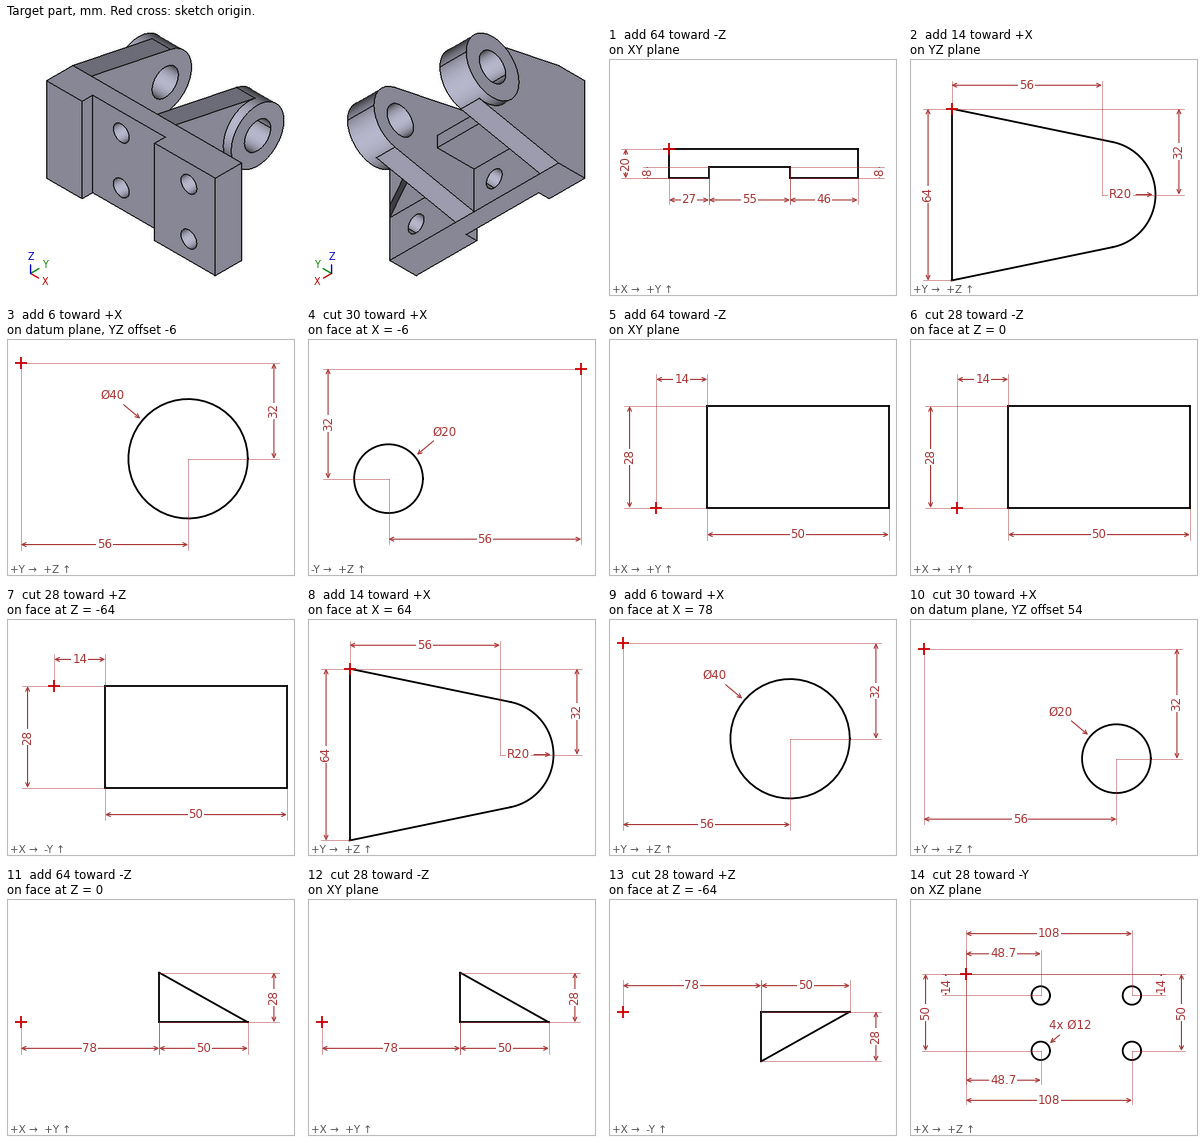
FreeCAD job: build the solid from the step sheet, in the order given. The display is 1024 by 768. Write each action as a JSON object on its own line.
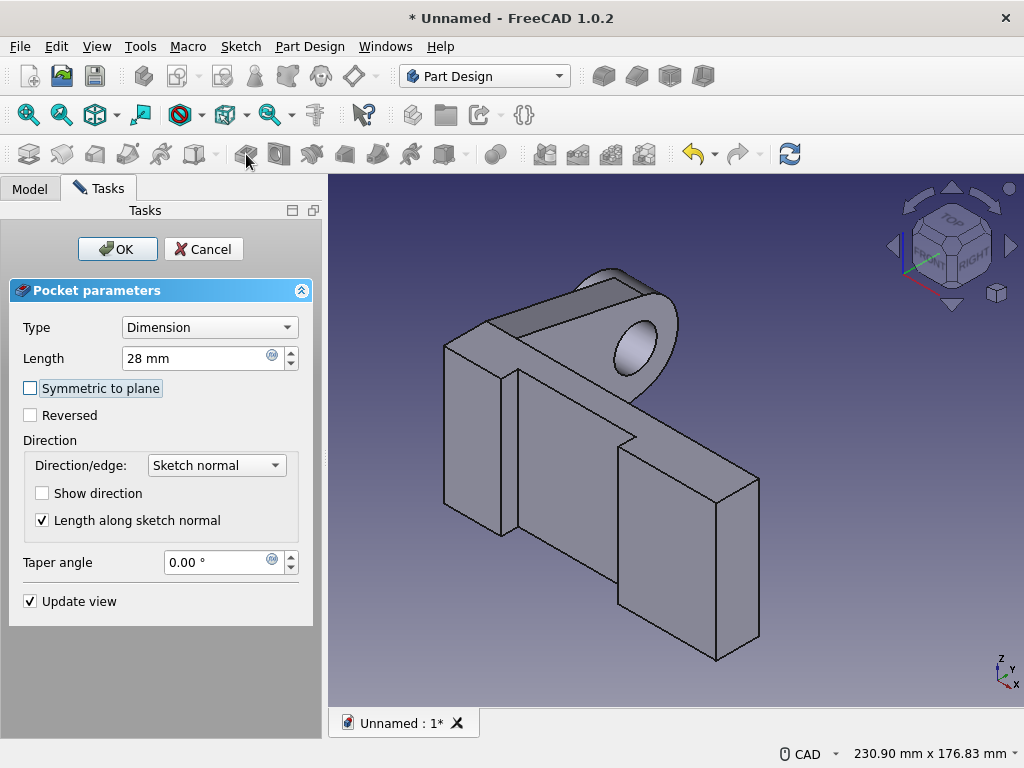
{"action": "left_click", "coordinate": [118, 249]}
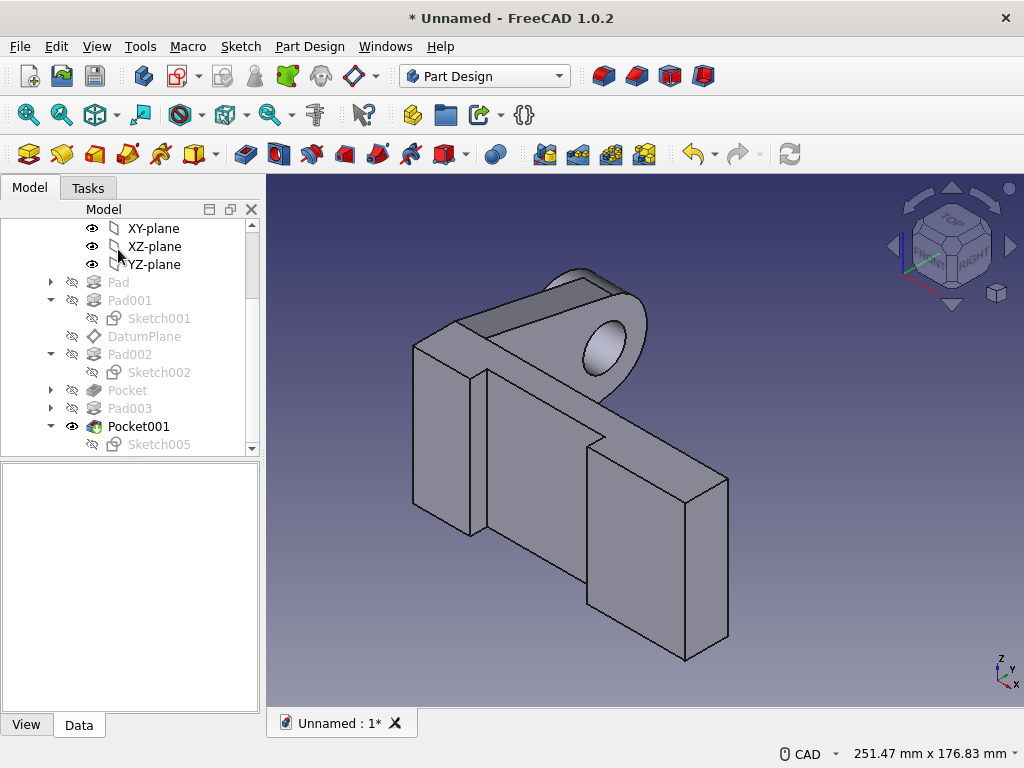
{"action": "key", "text": "5"}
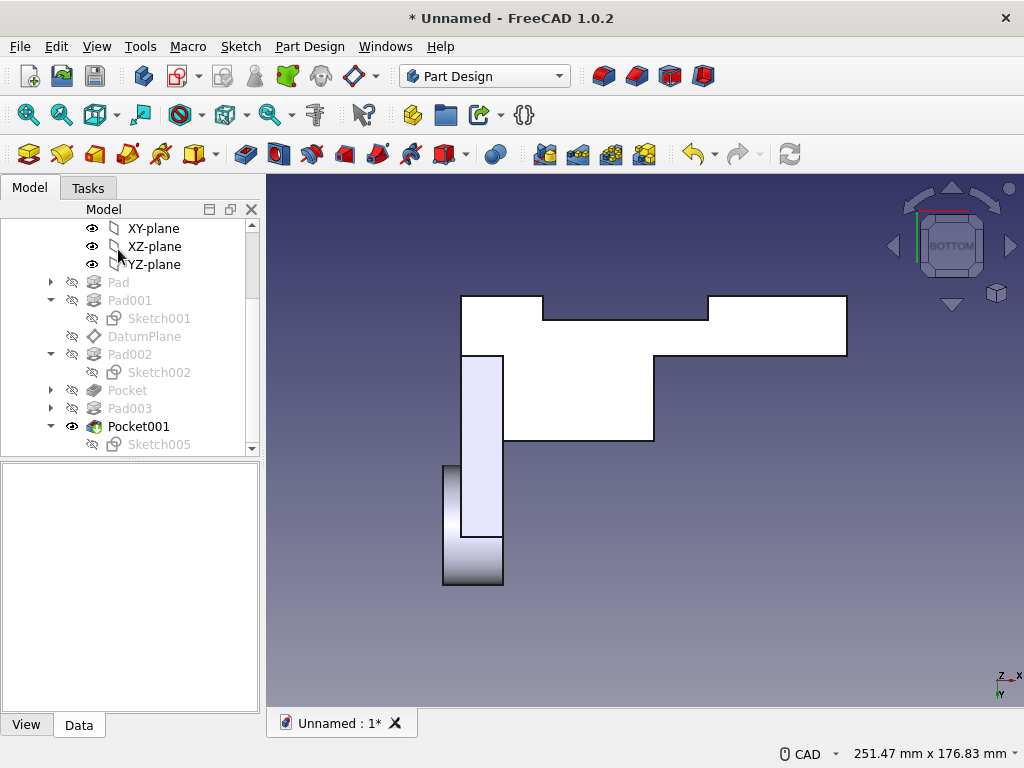
{"action": "left_click", "coordinate": [599, 388]}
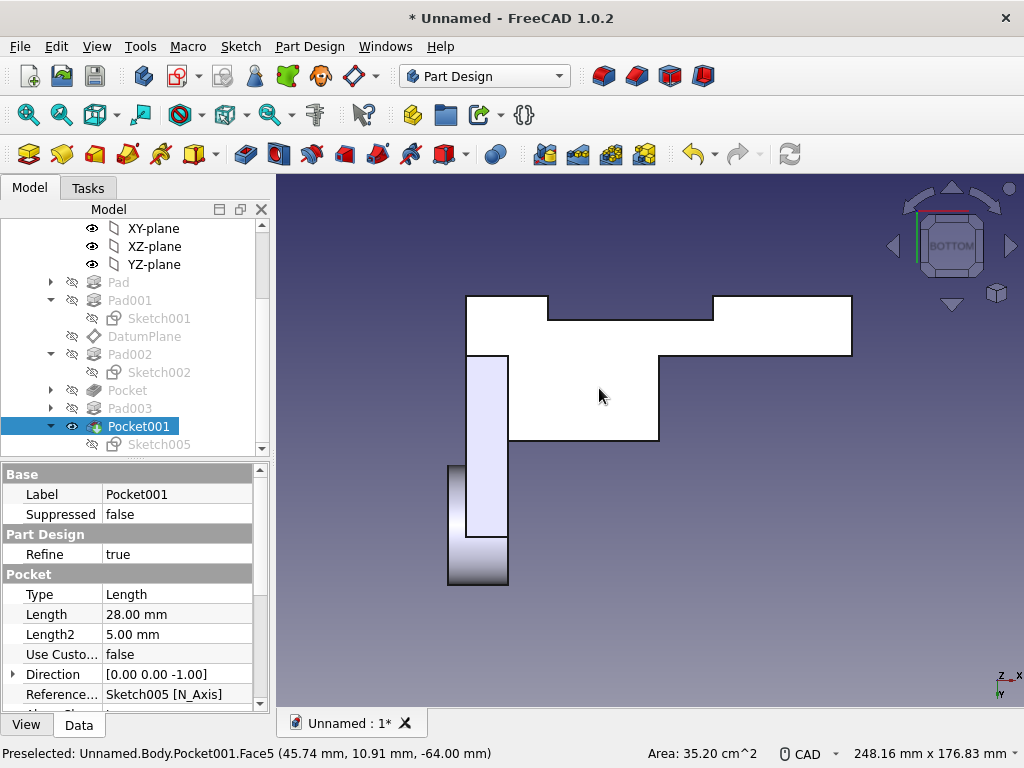
{"action": "left_click", "coordinate": [176, 76]}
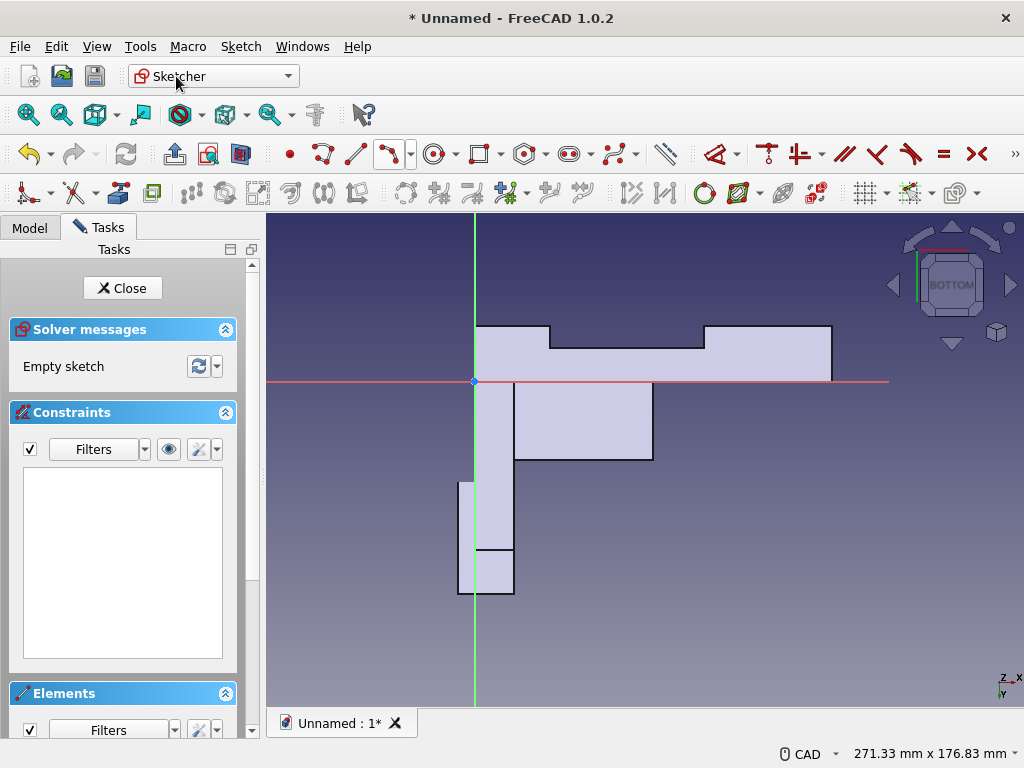
{"action": "scroll", "coordinate": [554, 389], "scroll_direction": "up", "scroll_amount": 4}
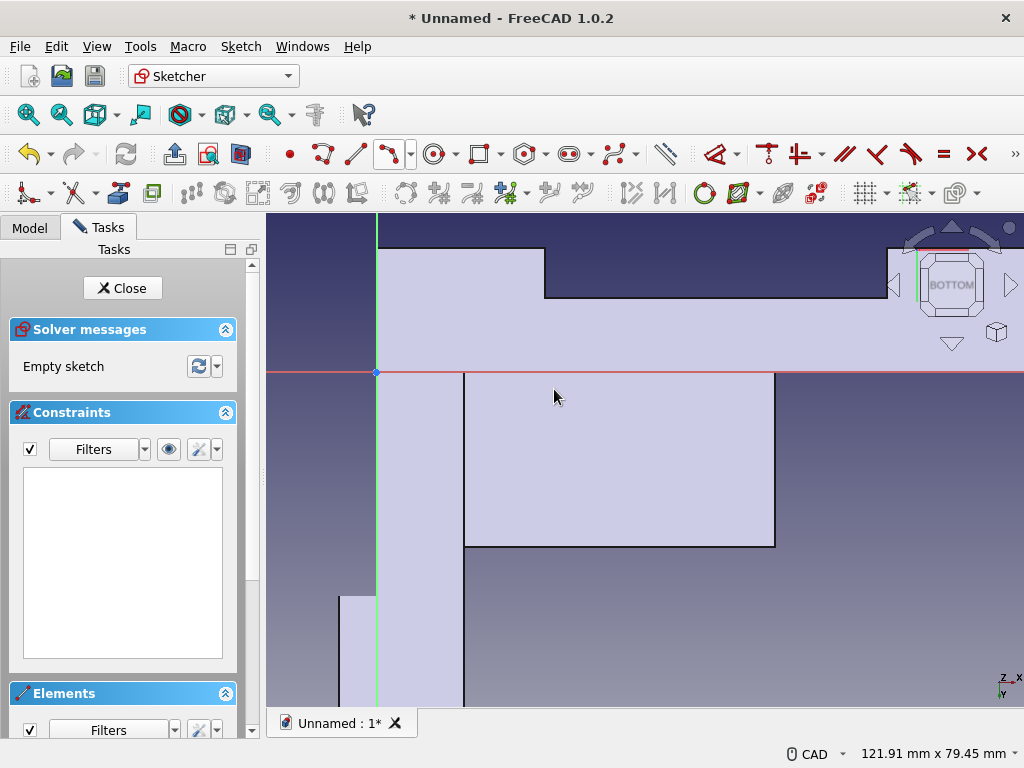
{"action": "left_click", "coordinate": [478, 154]}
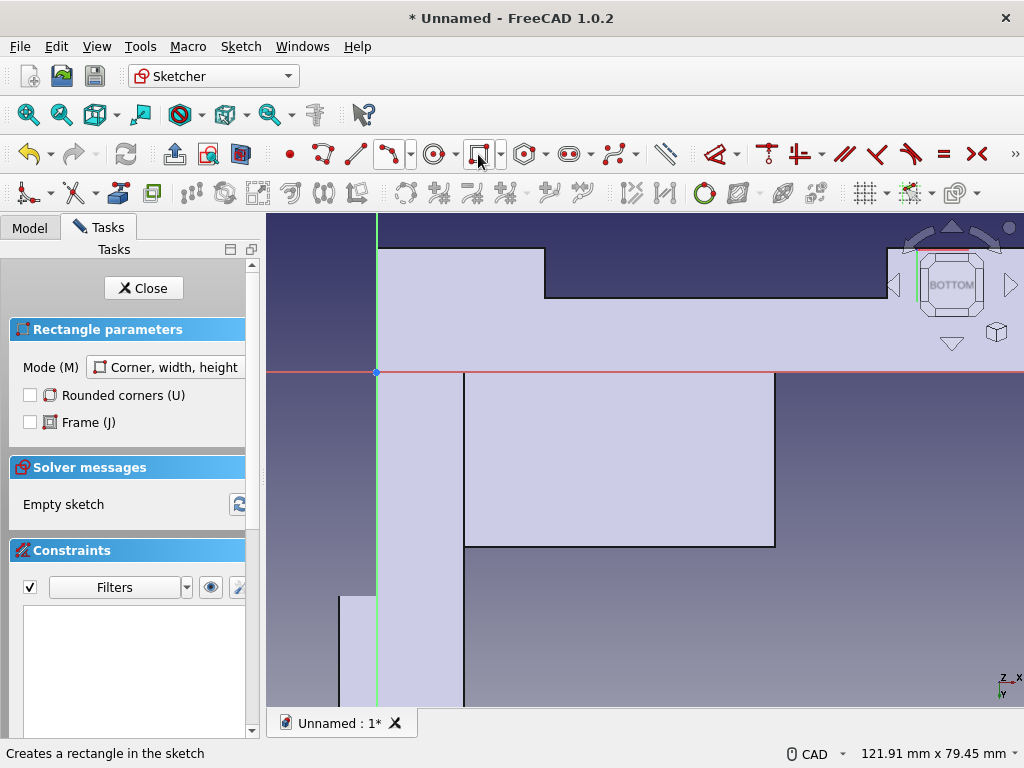
{"action": "left_click", "coordinate": [464, 372]}
{"action": "left_click", "coordinate": [775, 547]}
{"action": "key", "text": "Escape"}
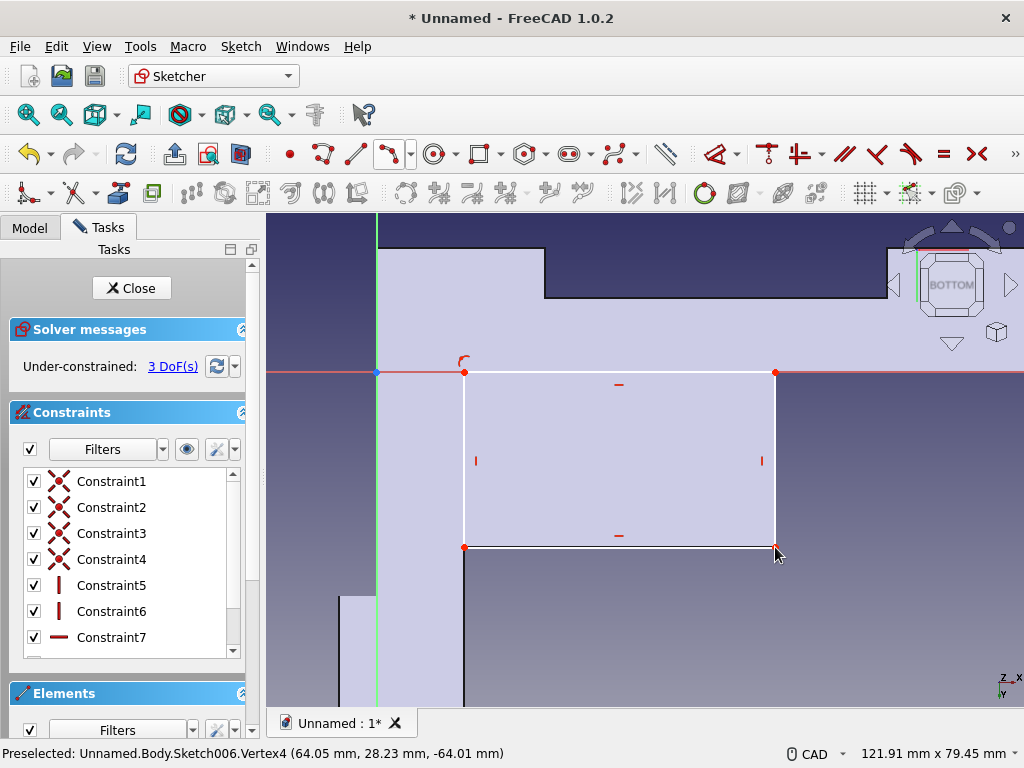
{"action": "left_click", "coordinate": [714, 154]}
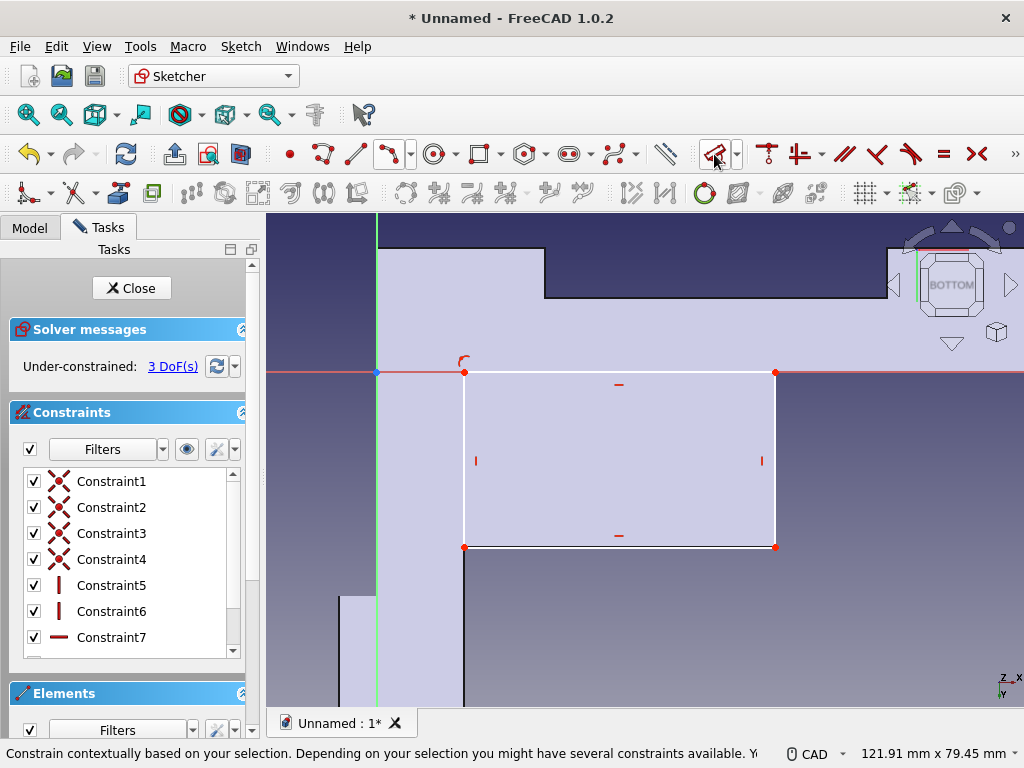
{"action": "left_click", "coordinate": [464, 425]}
{"action": "left_click", "coordinate": [430, 460]}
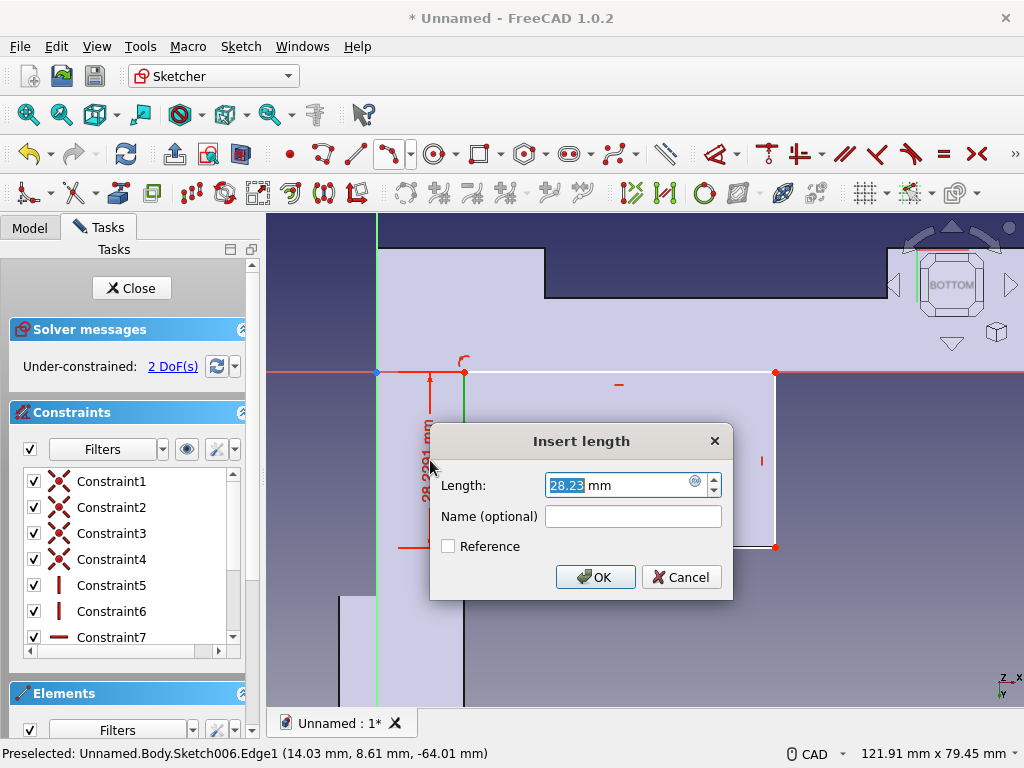
{"action": "type", "text": "28"}
{"action": "key", "text": "Return"}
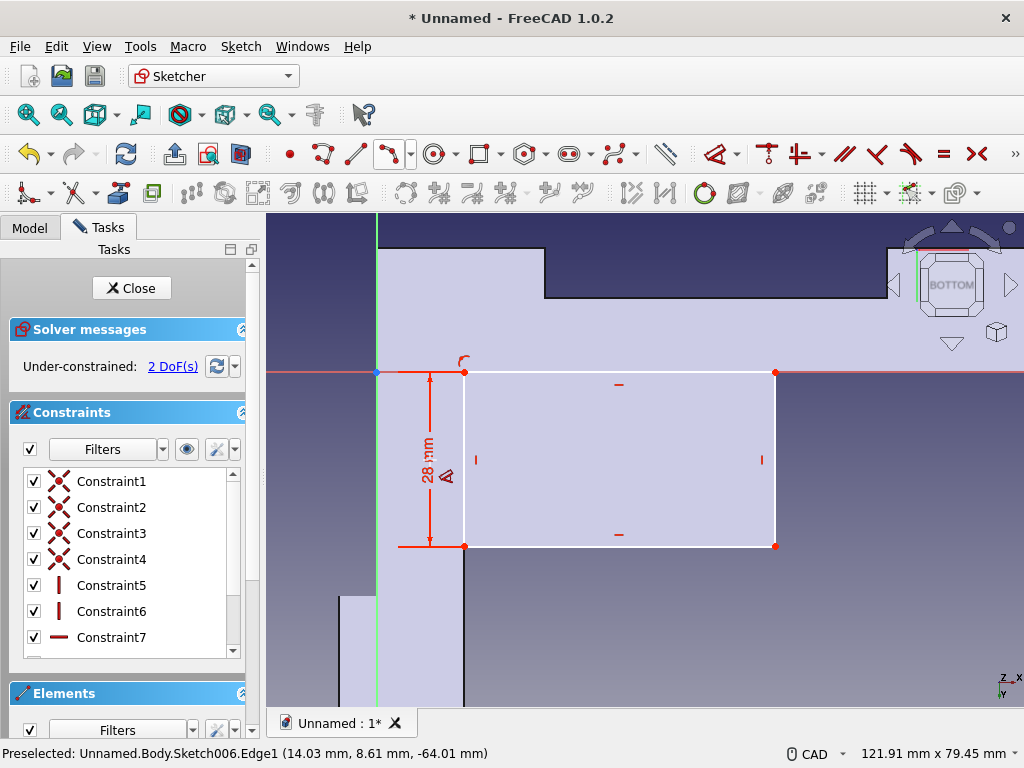
{"action": "left_click", "coordinate": [557, 547]}
{"action": "left_click", "coordinate": [620, 581]}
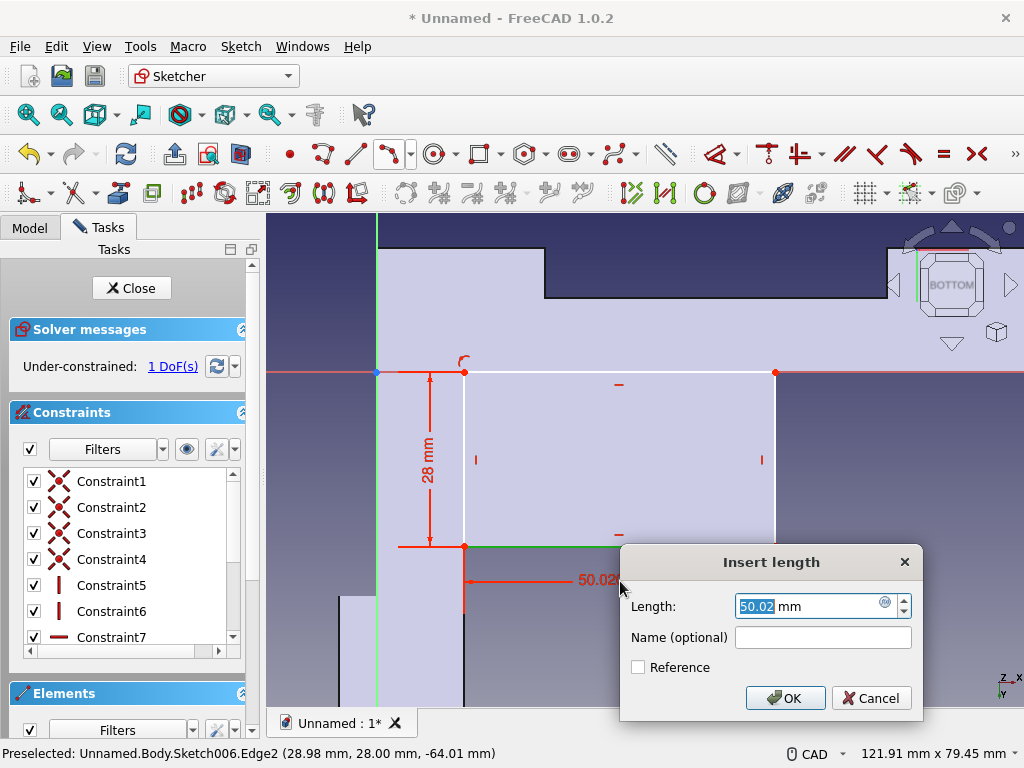
{"action": "type", "text": "50"}
{"action": "key", "text": "Return"}